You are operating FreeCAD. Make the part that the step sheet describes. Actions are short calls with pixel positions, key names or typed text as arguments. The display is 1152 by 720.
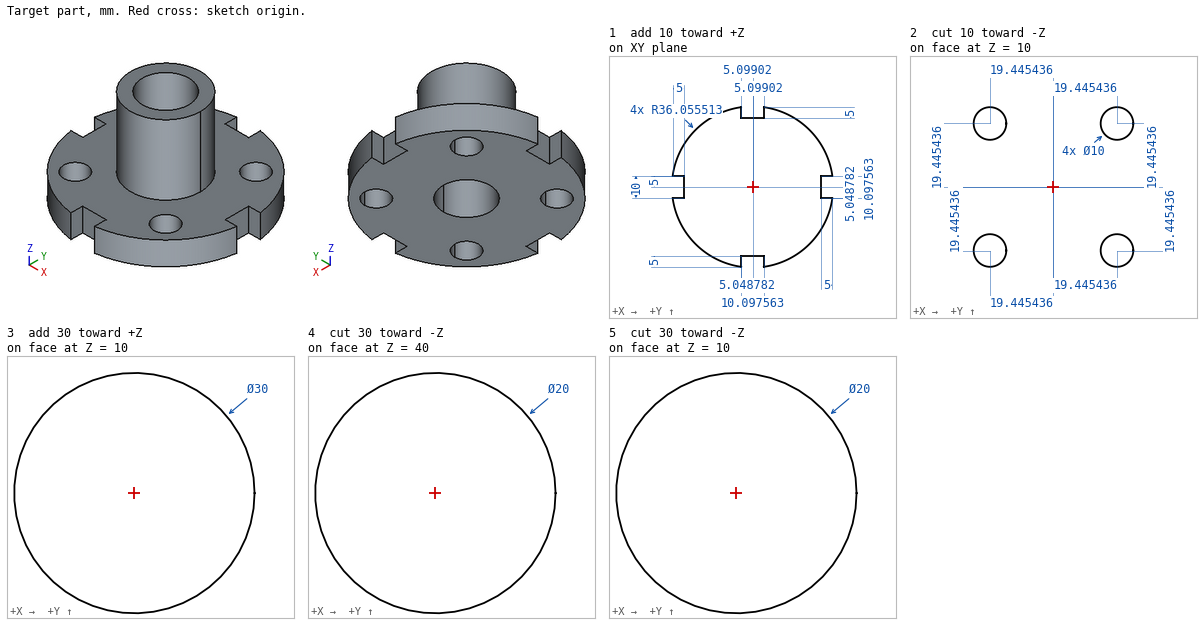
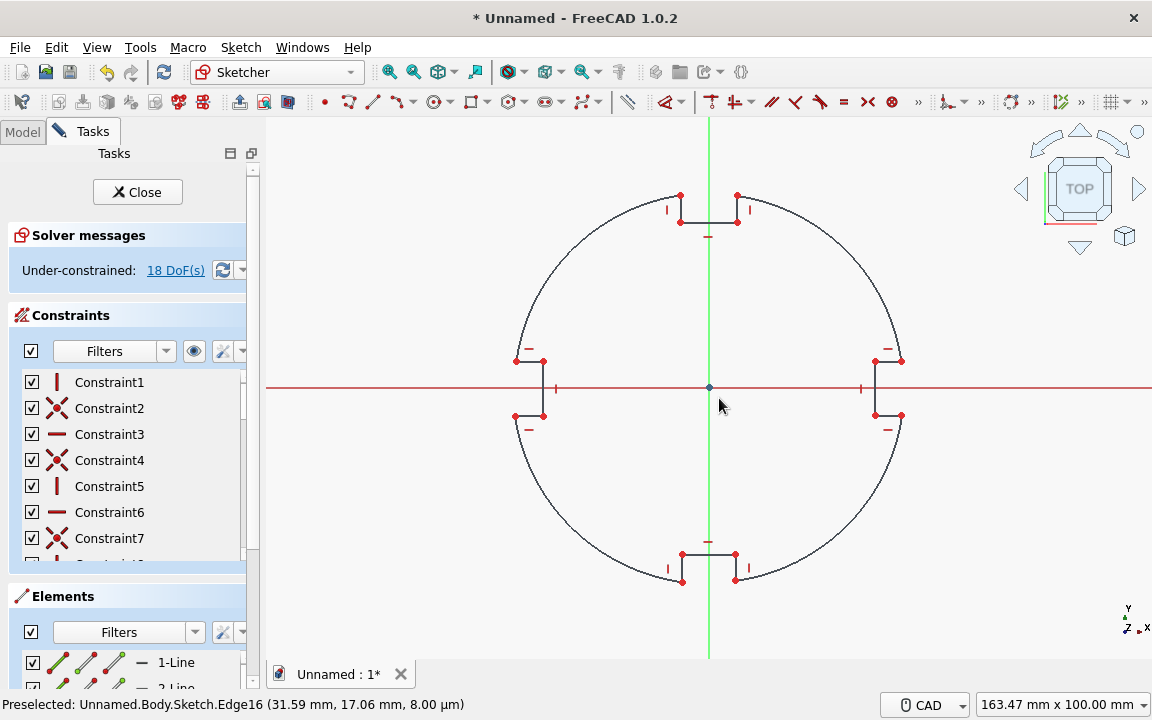
key(c)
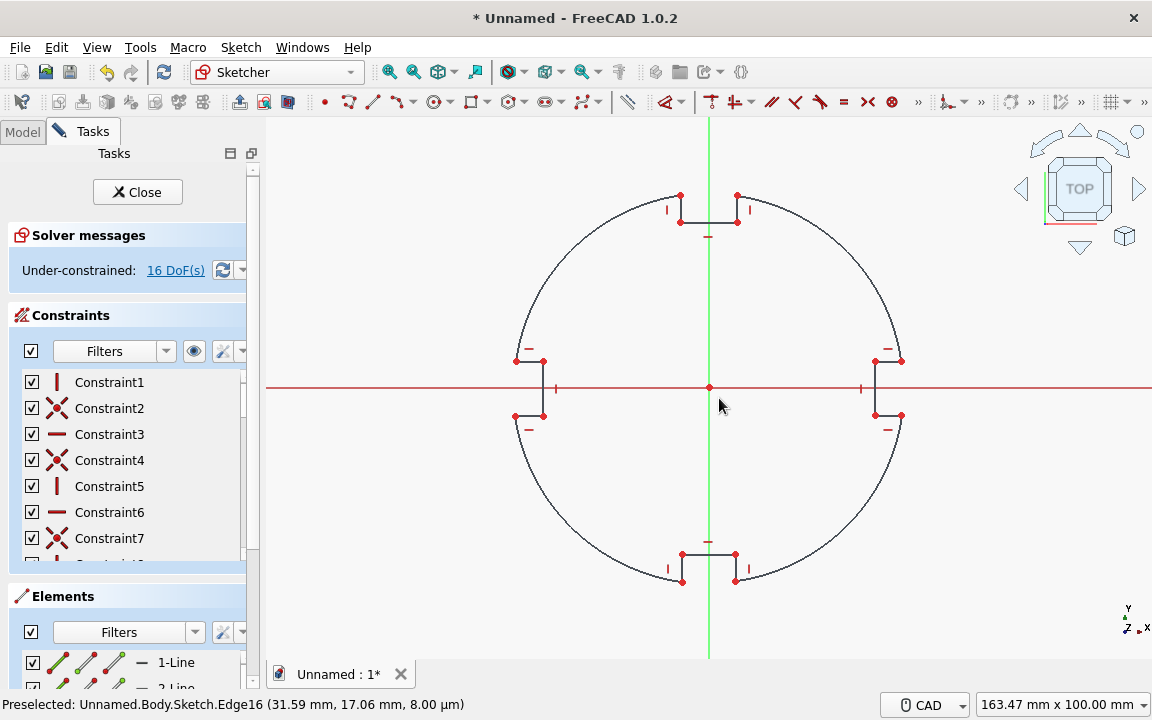
click(610, 220)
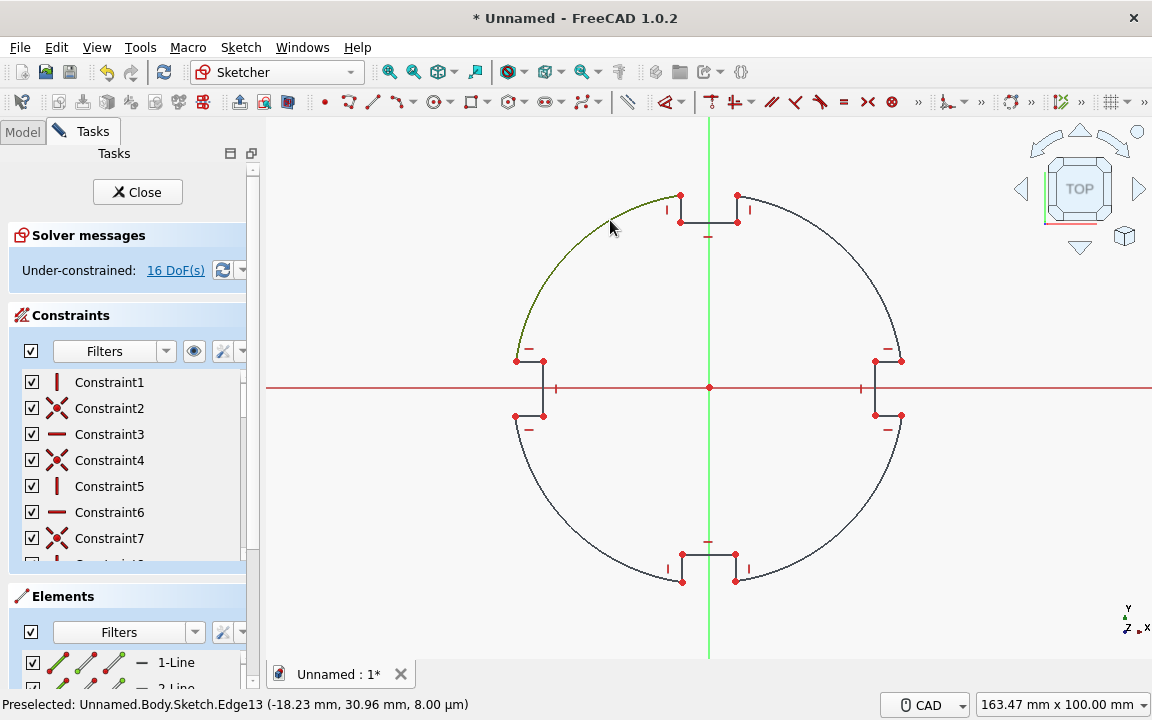
click(540, 487)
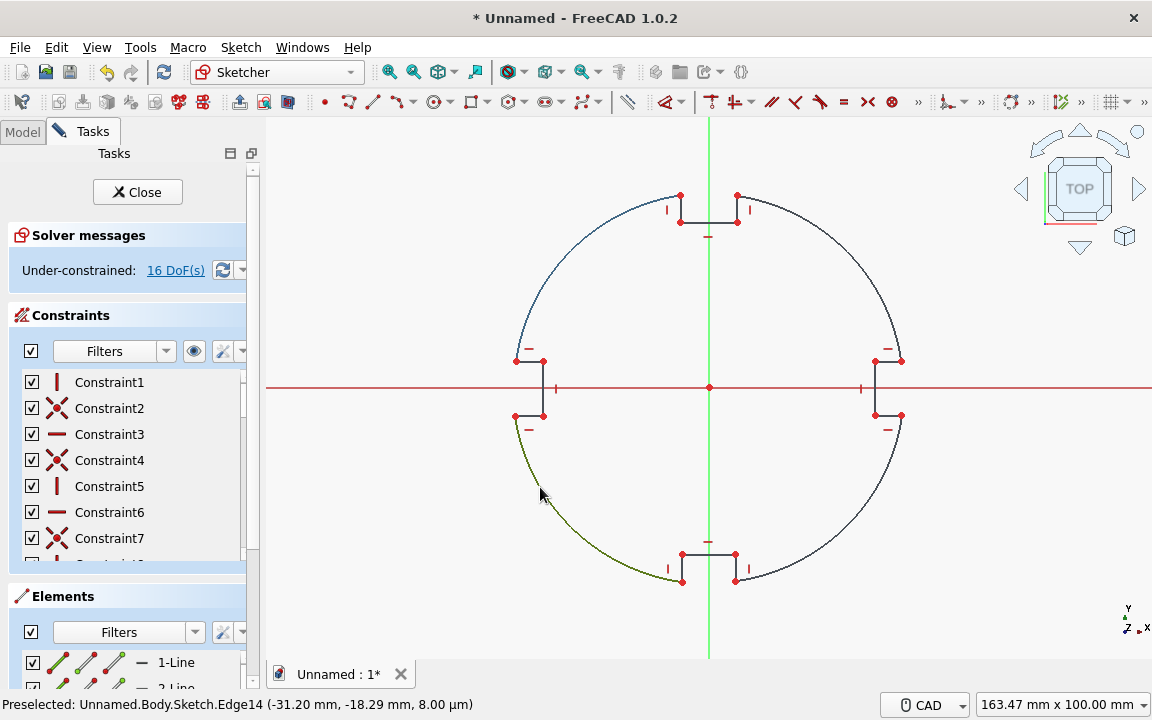
click(807, 557)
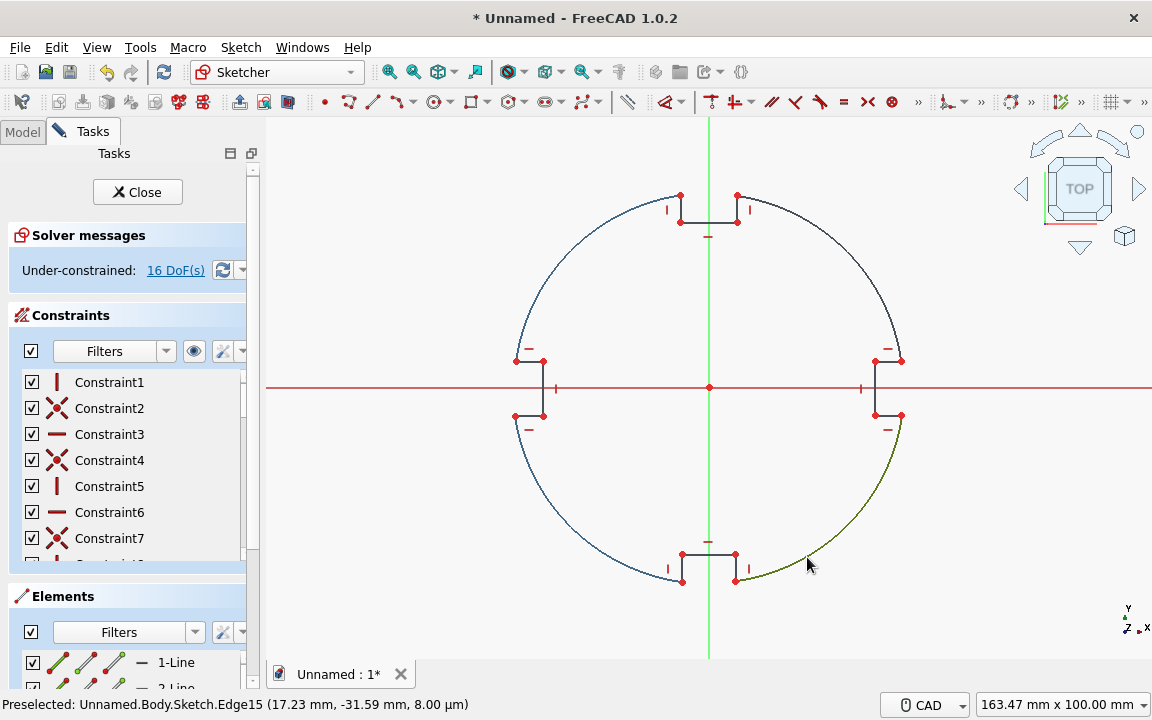
click(877, 291)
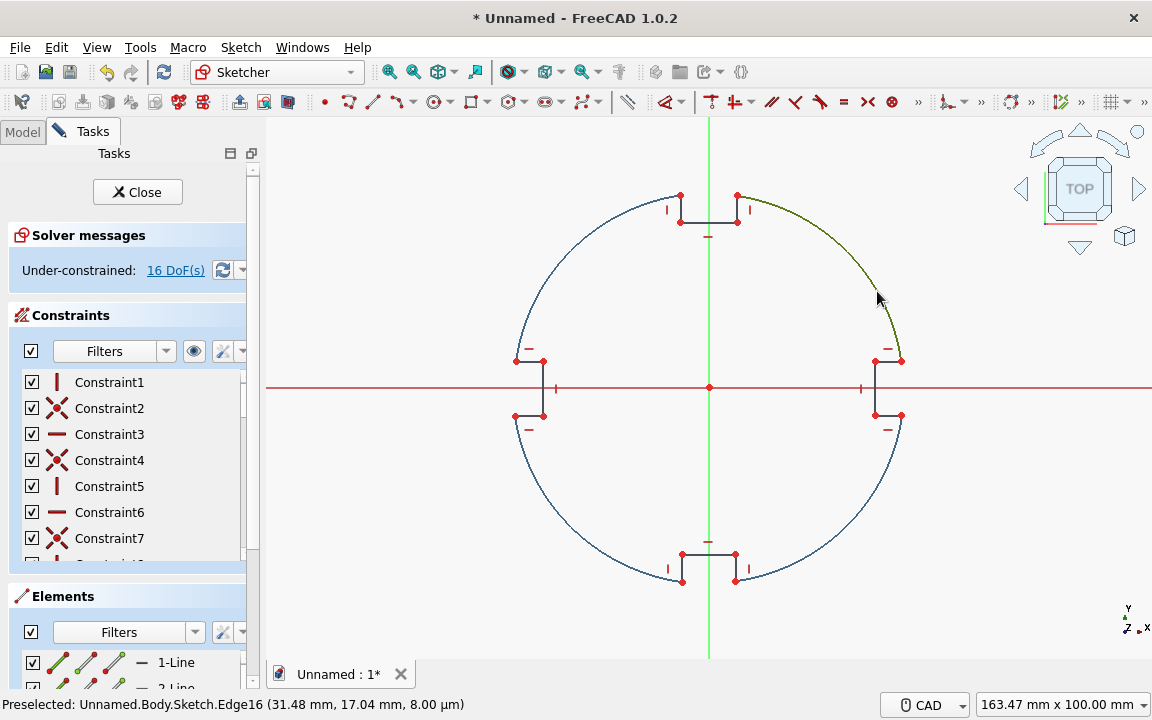
key(e)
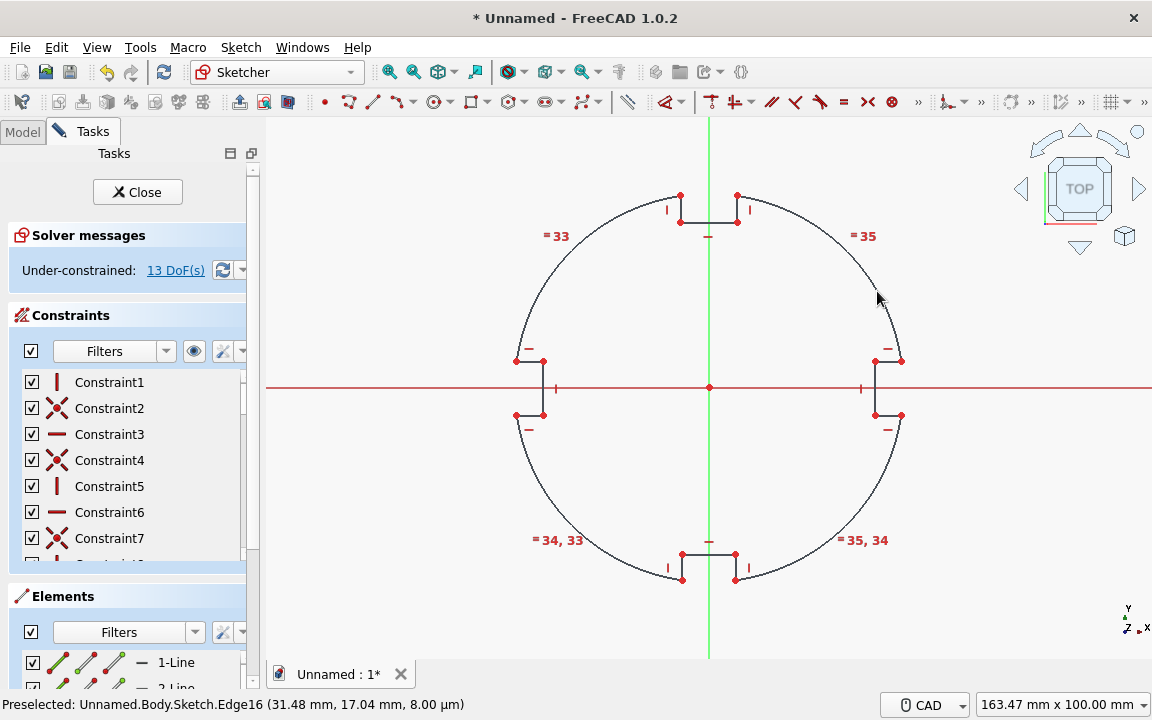
key(d)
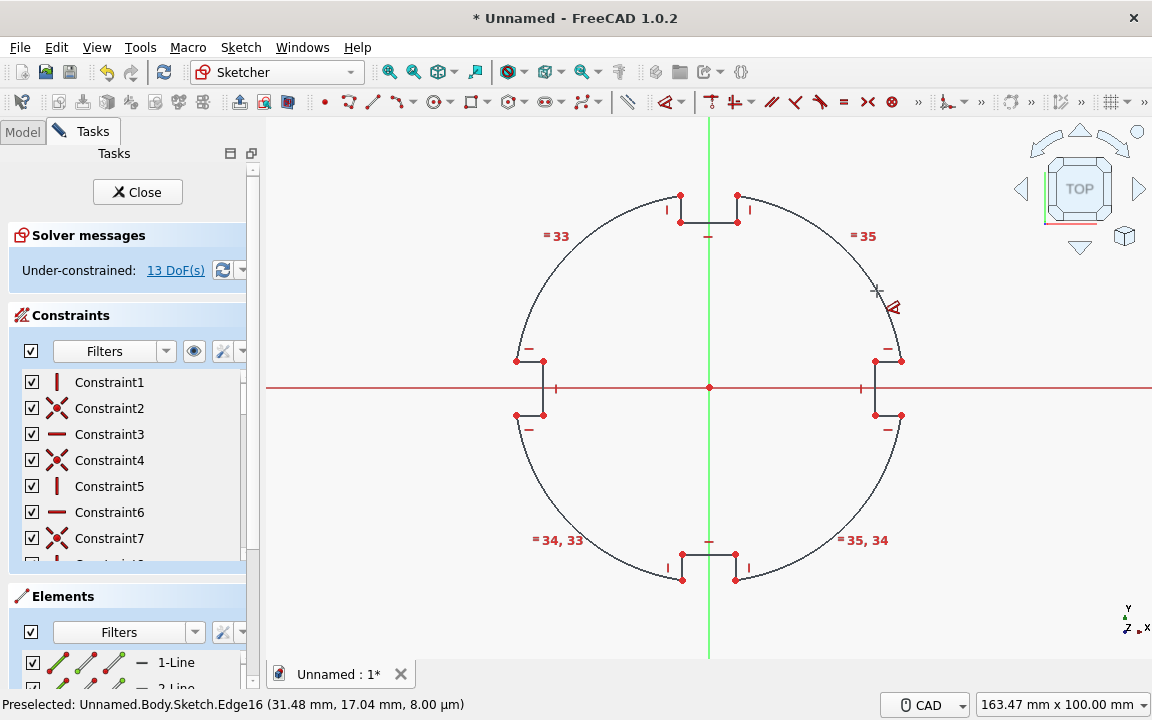
click(610, 221)
click(594, 193)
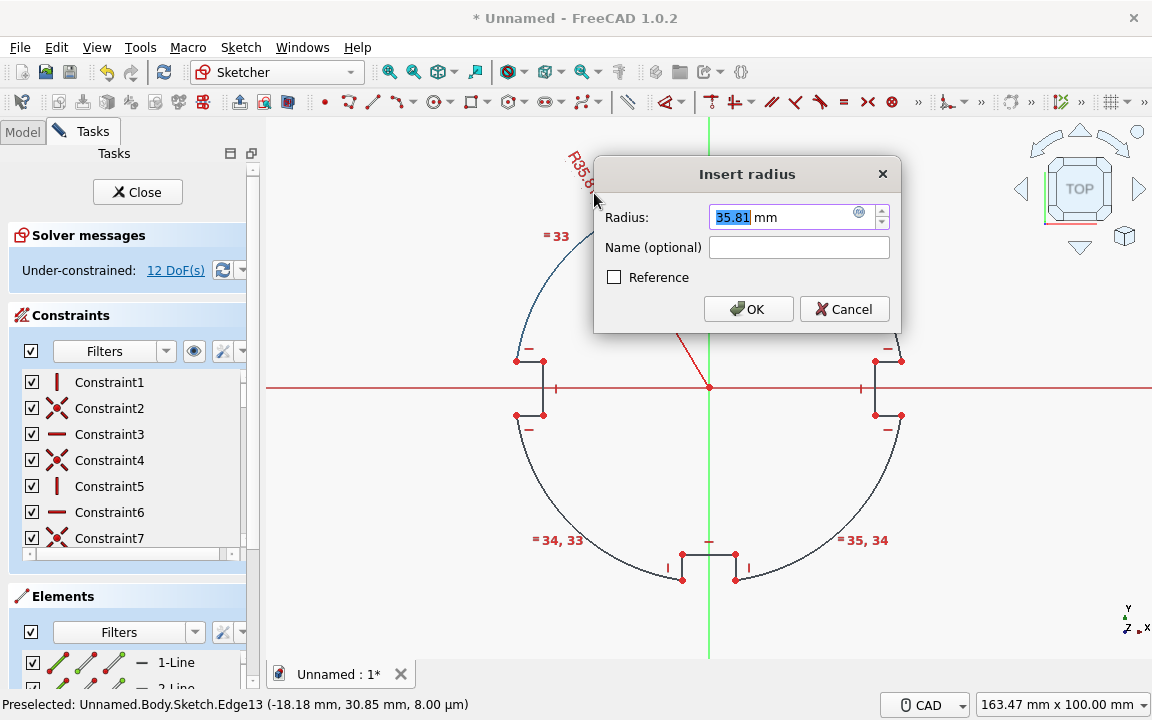
text(36.055513)
key(Return)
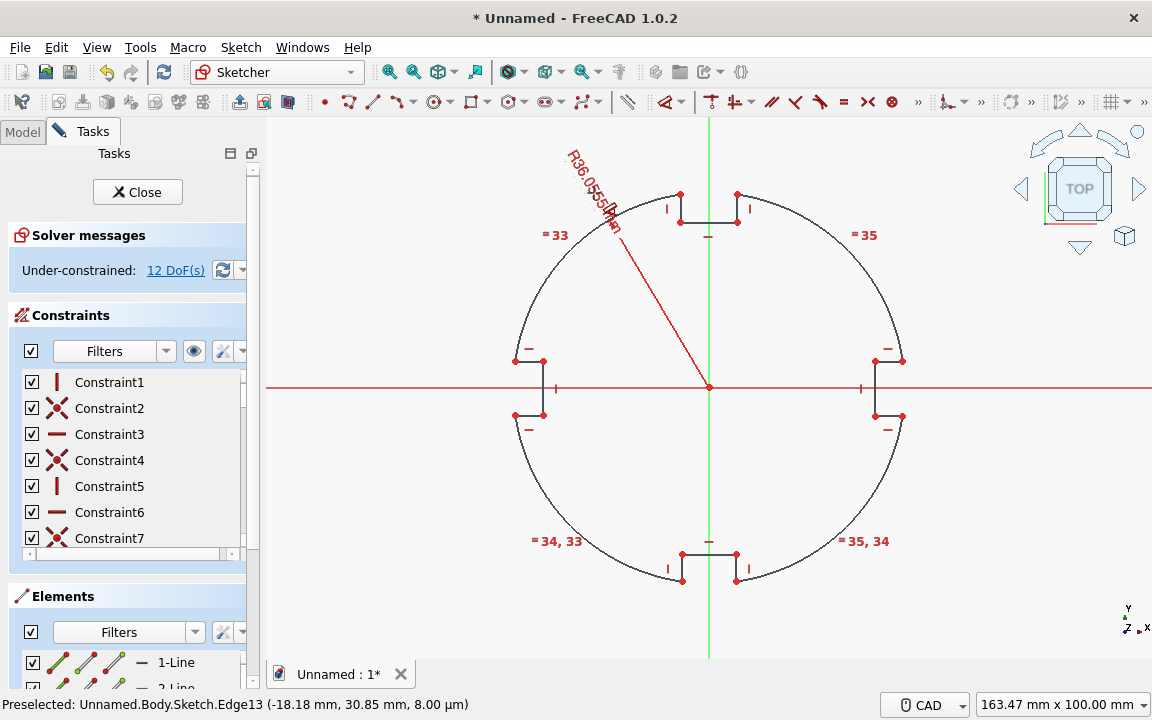
scroll(737, 206, up, 2)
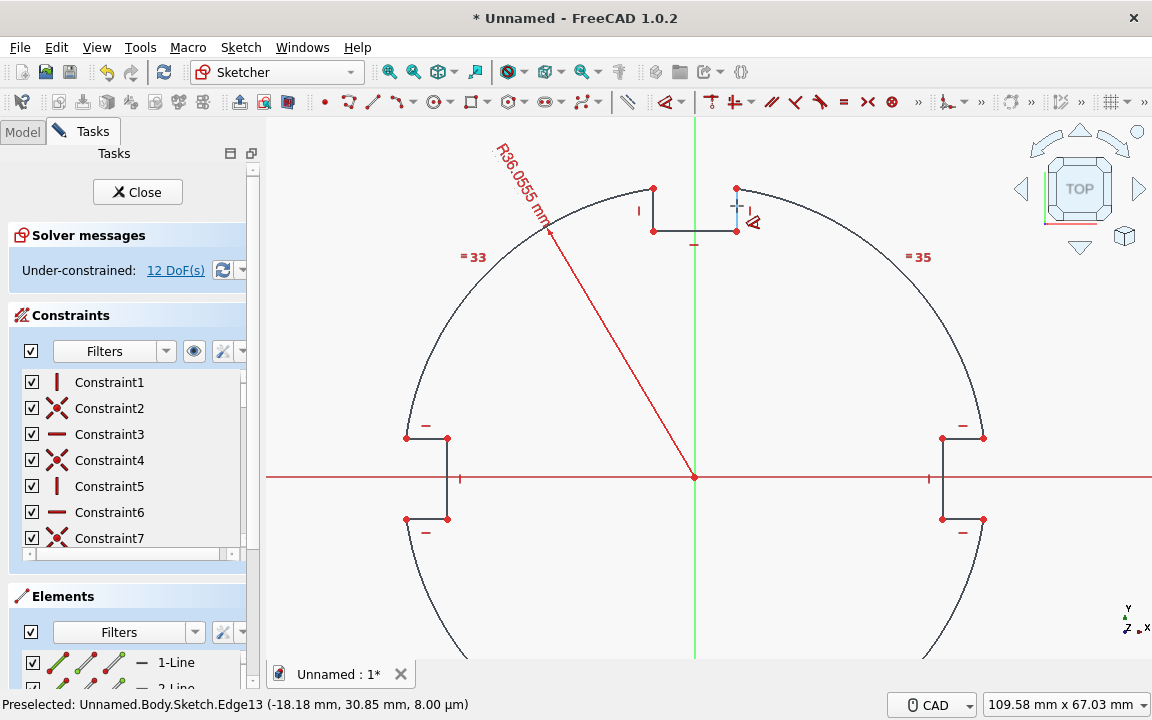
click(737, 206)
click(771, 210)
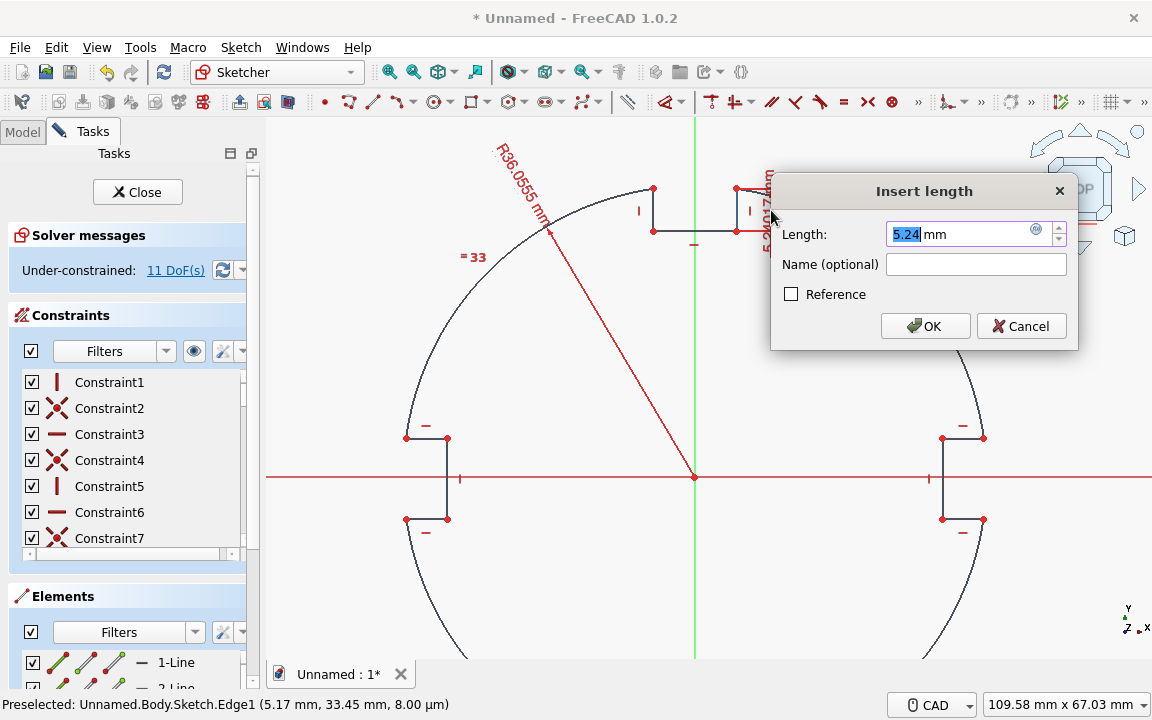
text(5)
key(Return)